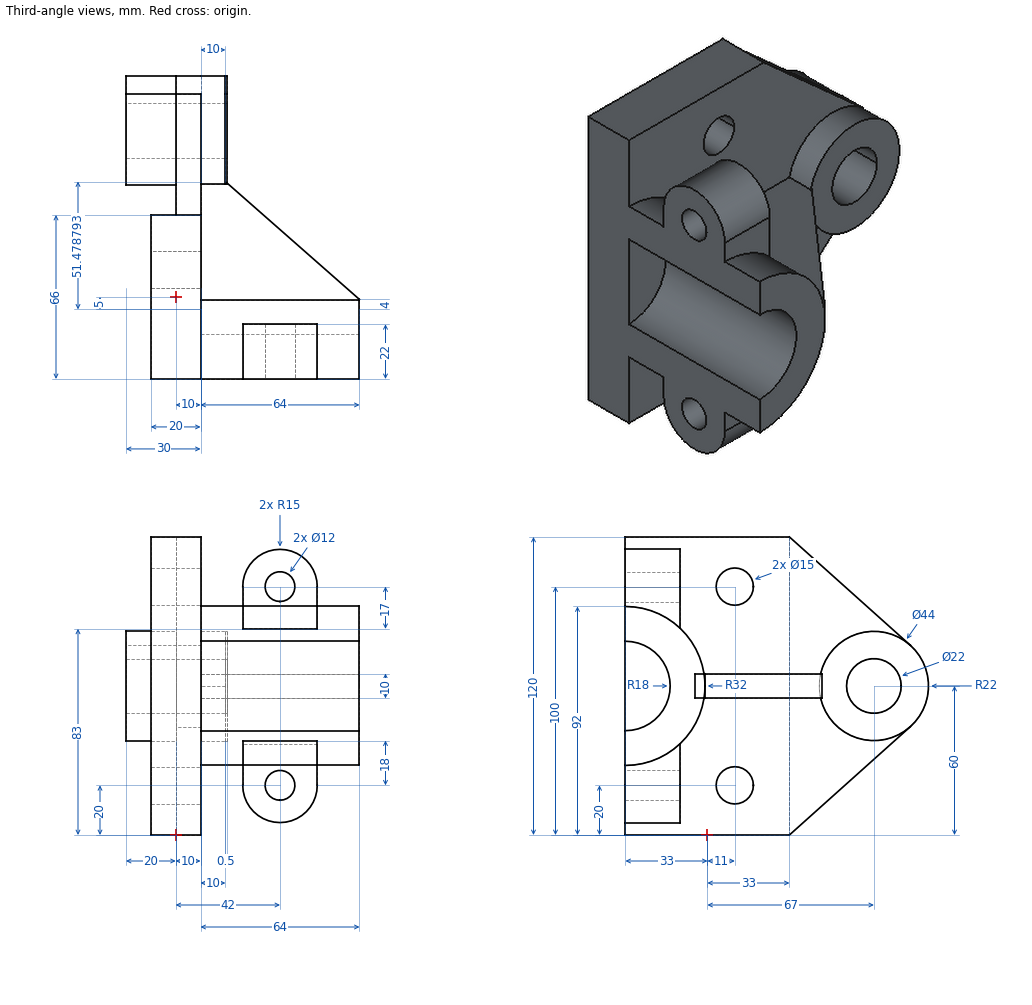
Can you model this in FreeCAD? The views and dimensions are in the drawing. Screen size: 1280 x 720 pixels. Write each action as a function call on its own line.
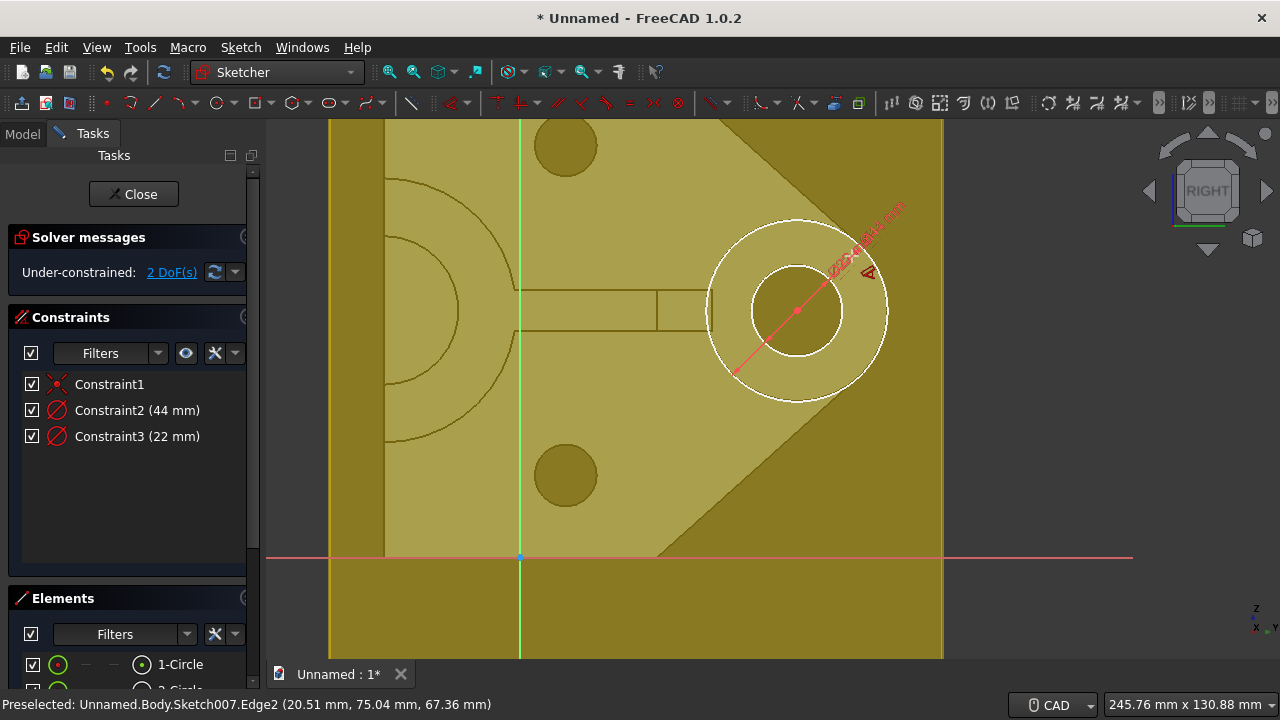
click(797, 311)
click(659, 592)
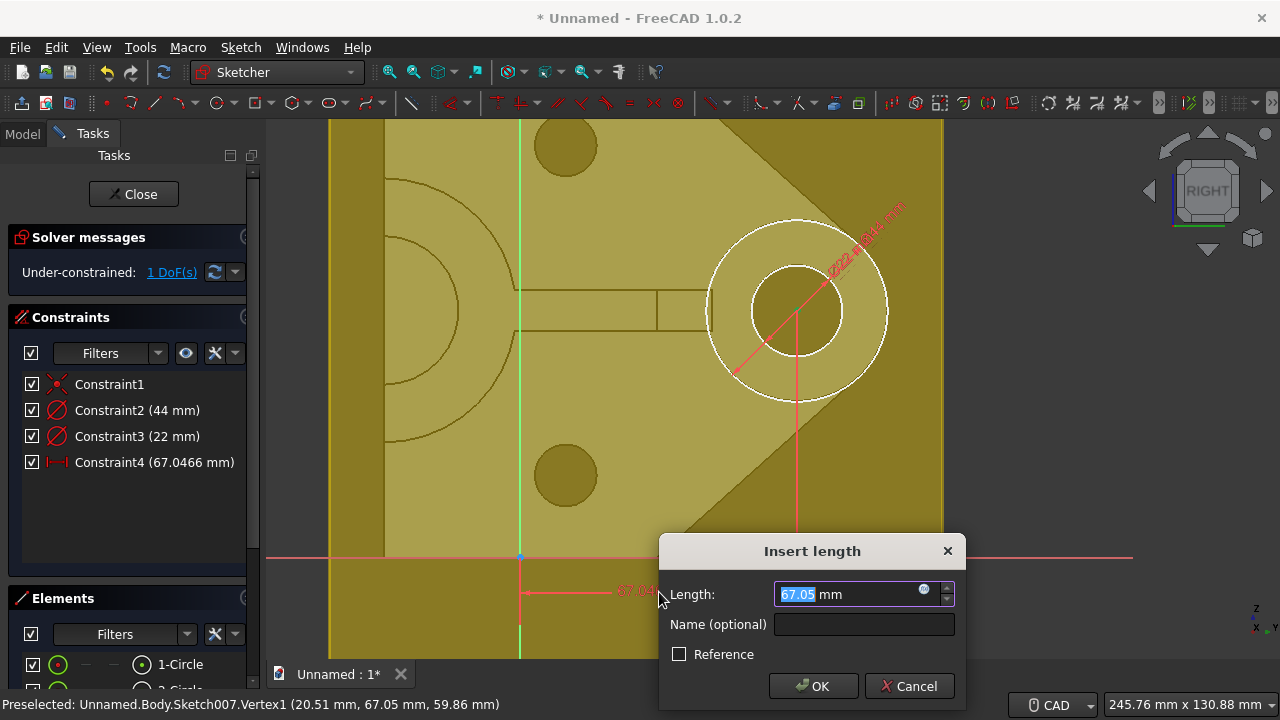
text(67)
key(Return)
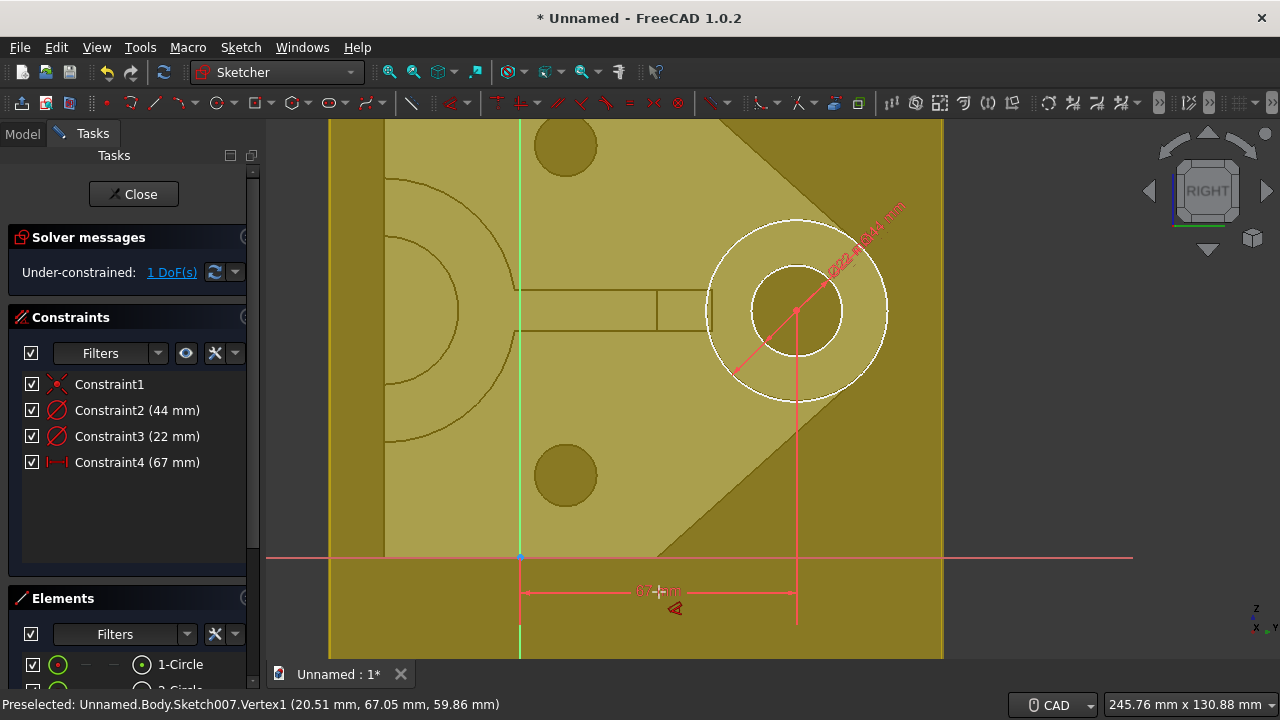
click(797, 311)
click(486, 434)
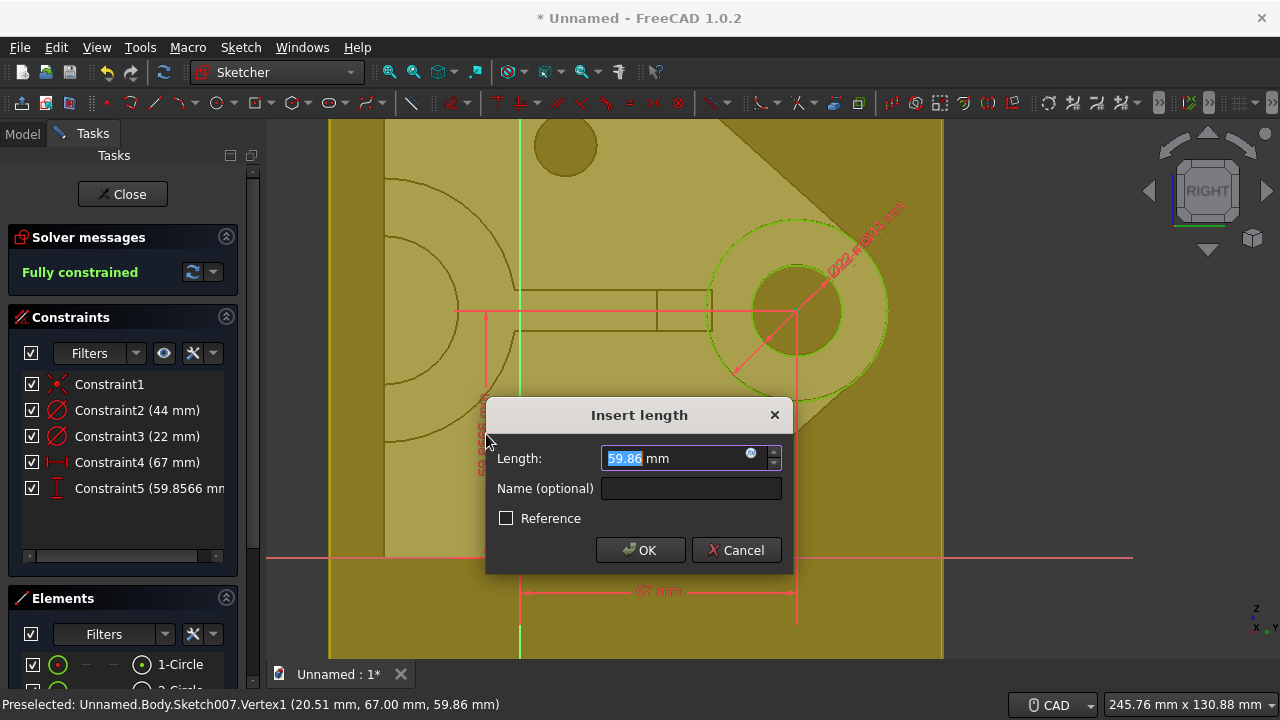
text(60)
key(Return)
key(Escape)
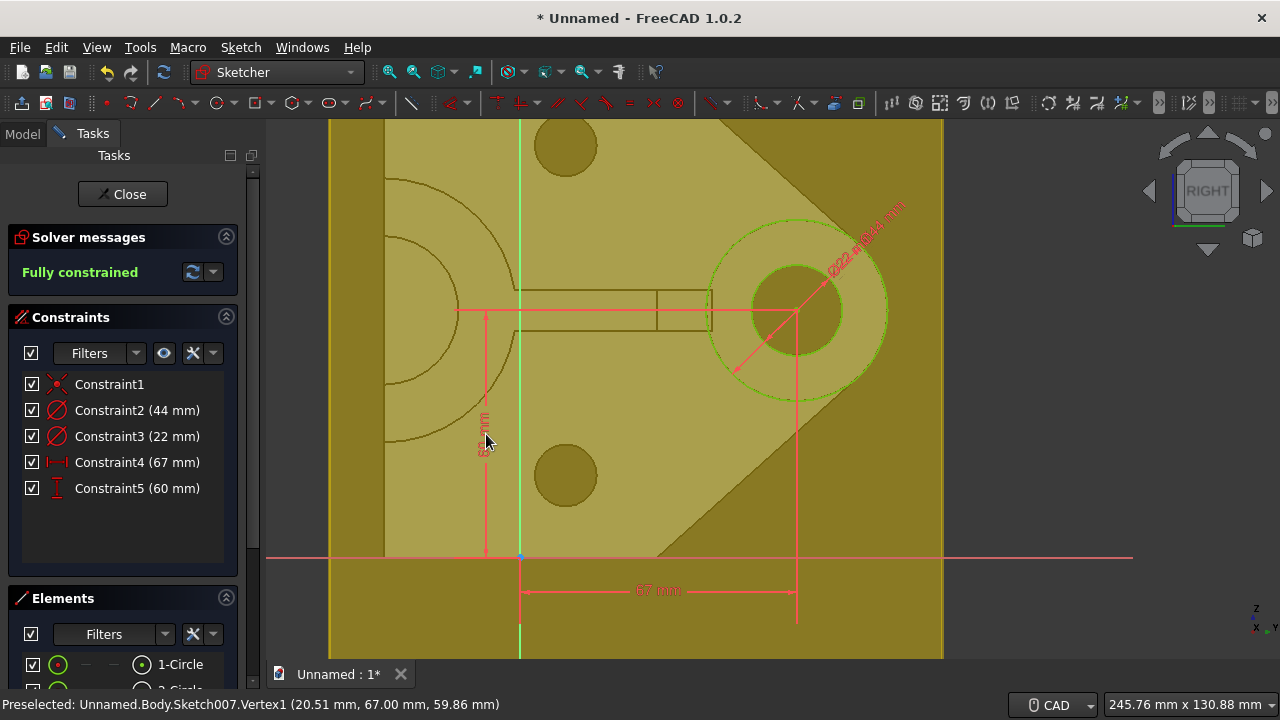
click(123, 194)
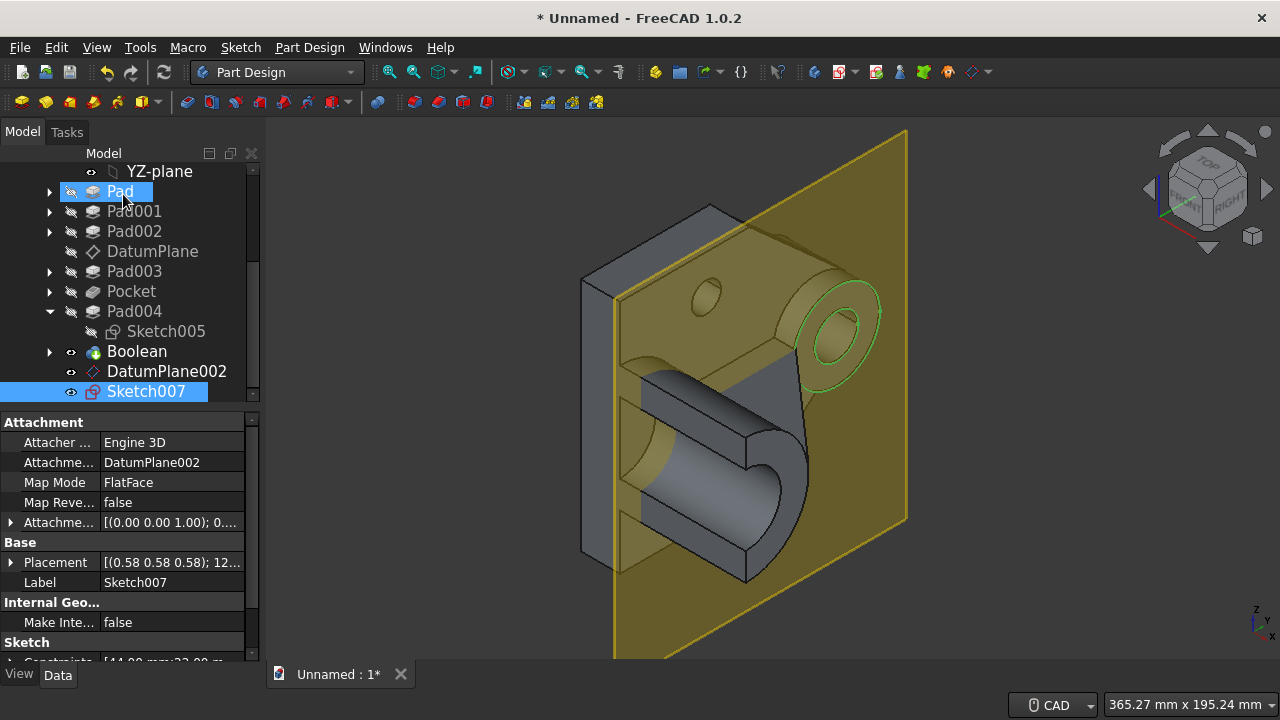
click(22, 102)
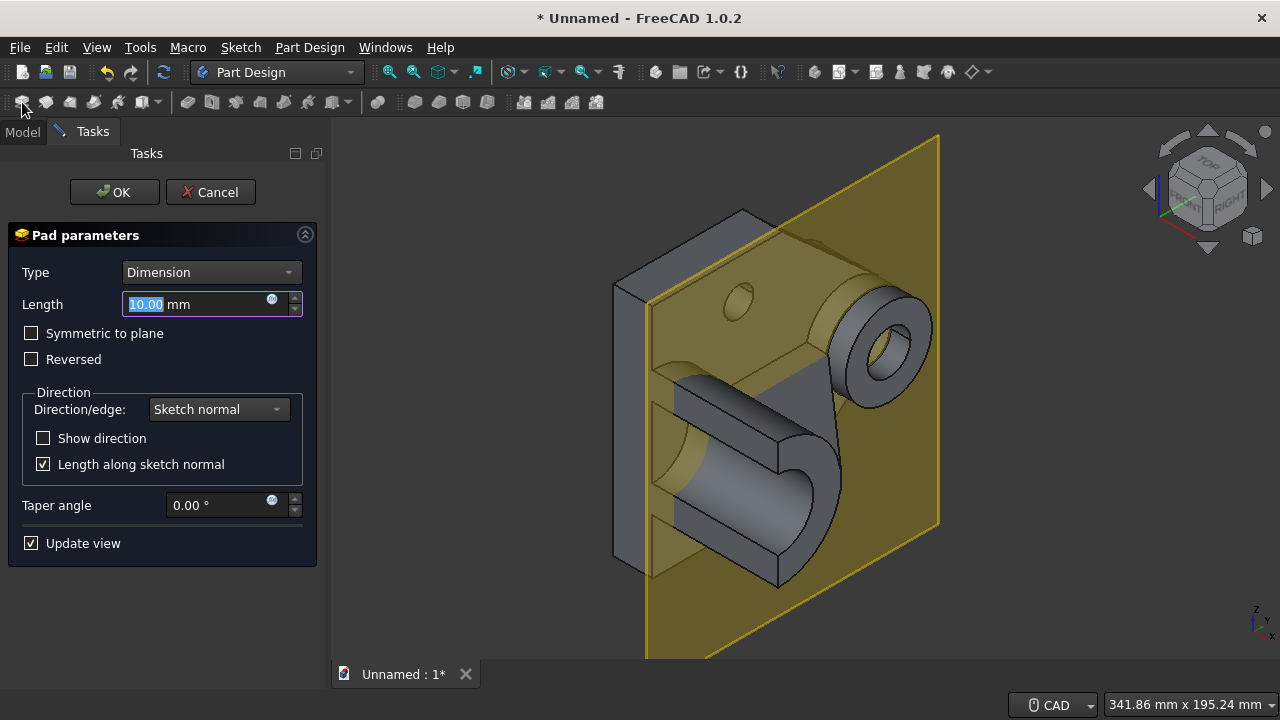
text(0.5)
key(Tab)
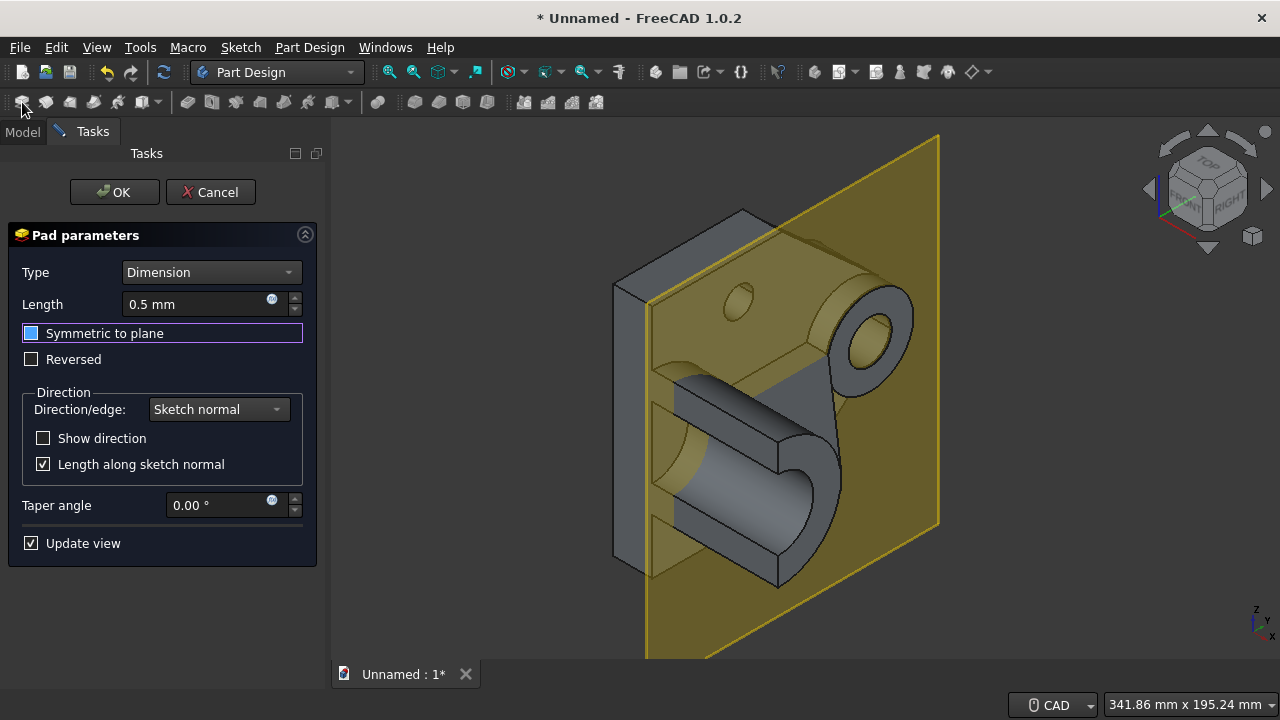
click(30, 359)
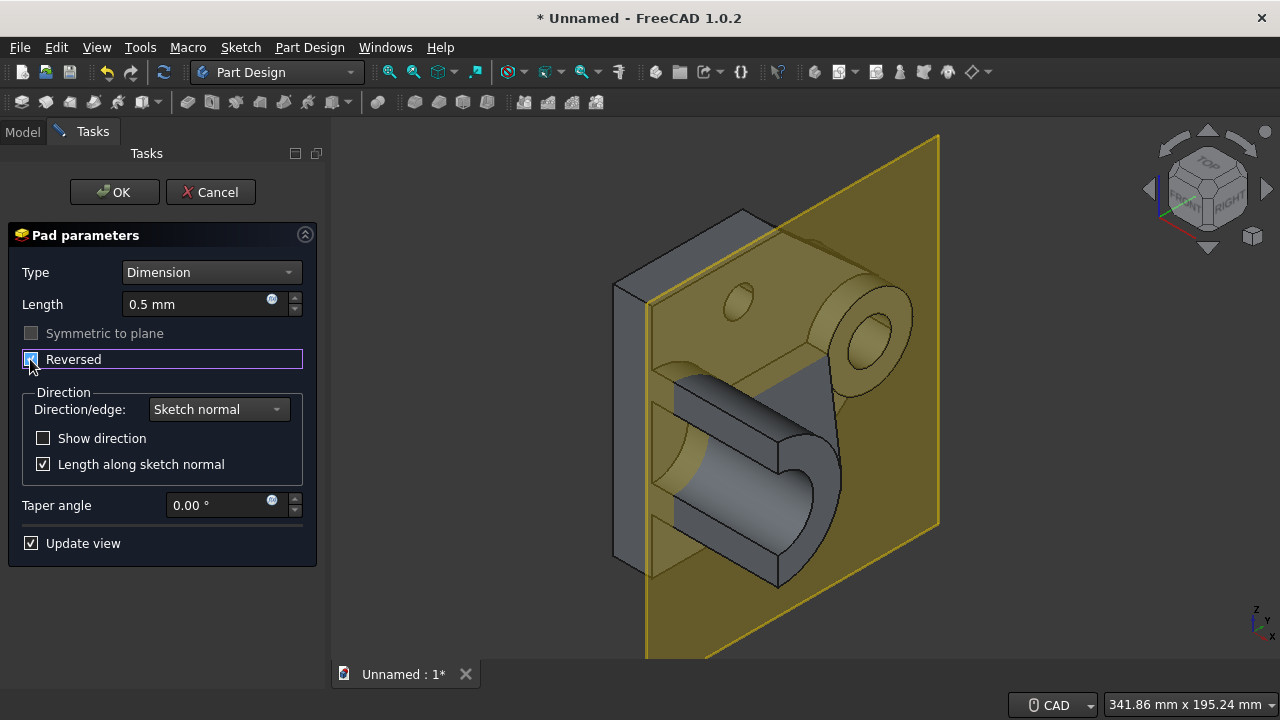
click(115, 192)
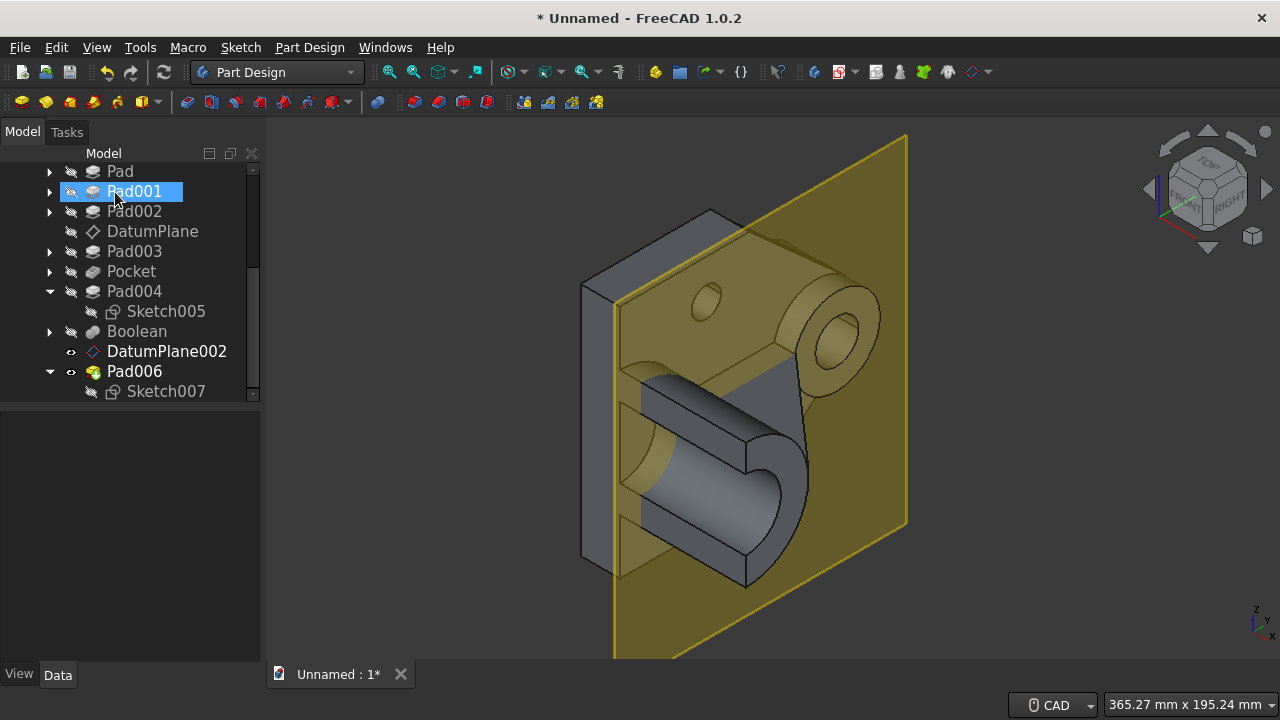
click(116, 352)
key(space)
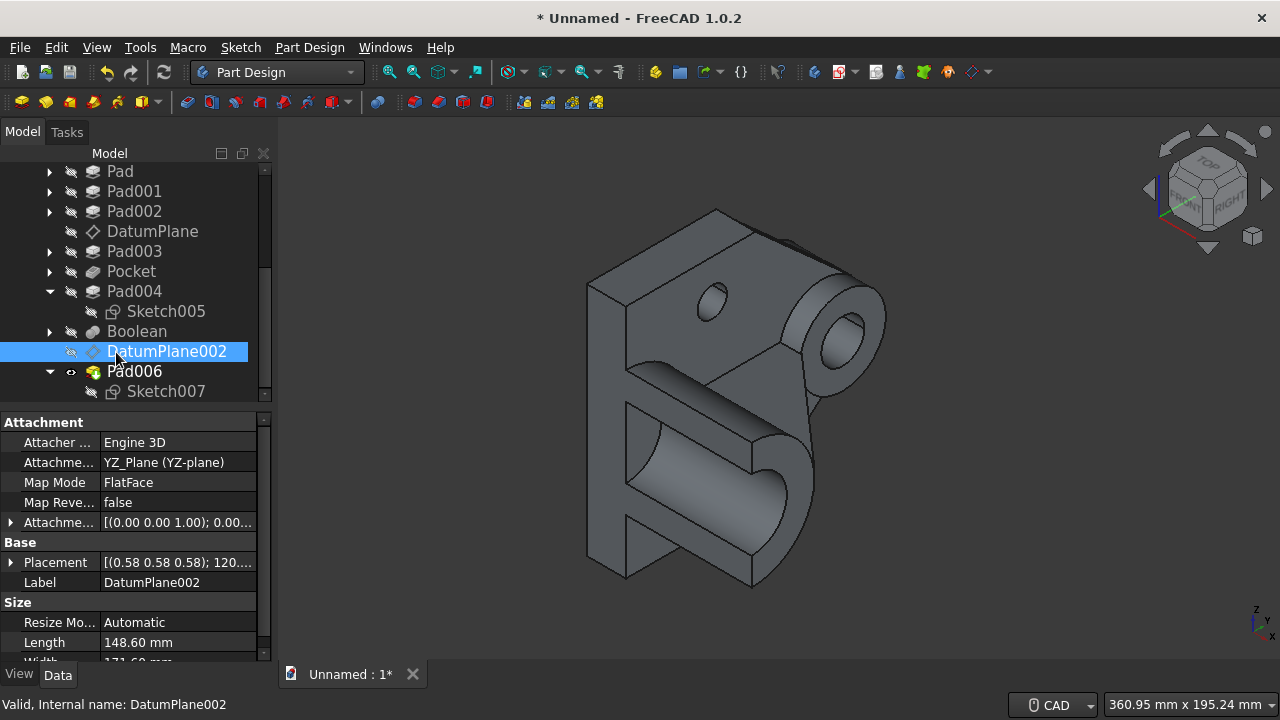
click(598, 309)